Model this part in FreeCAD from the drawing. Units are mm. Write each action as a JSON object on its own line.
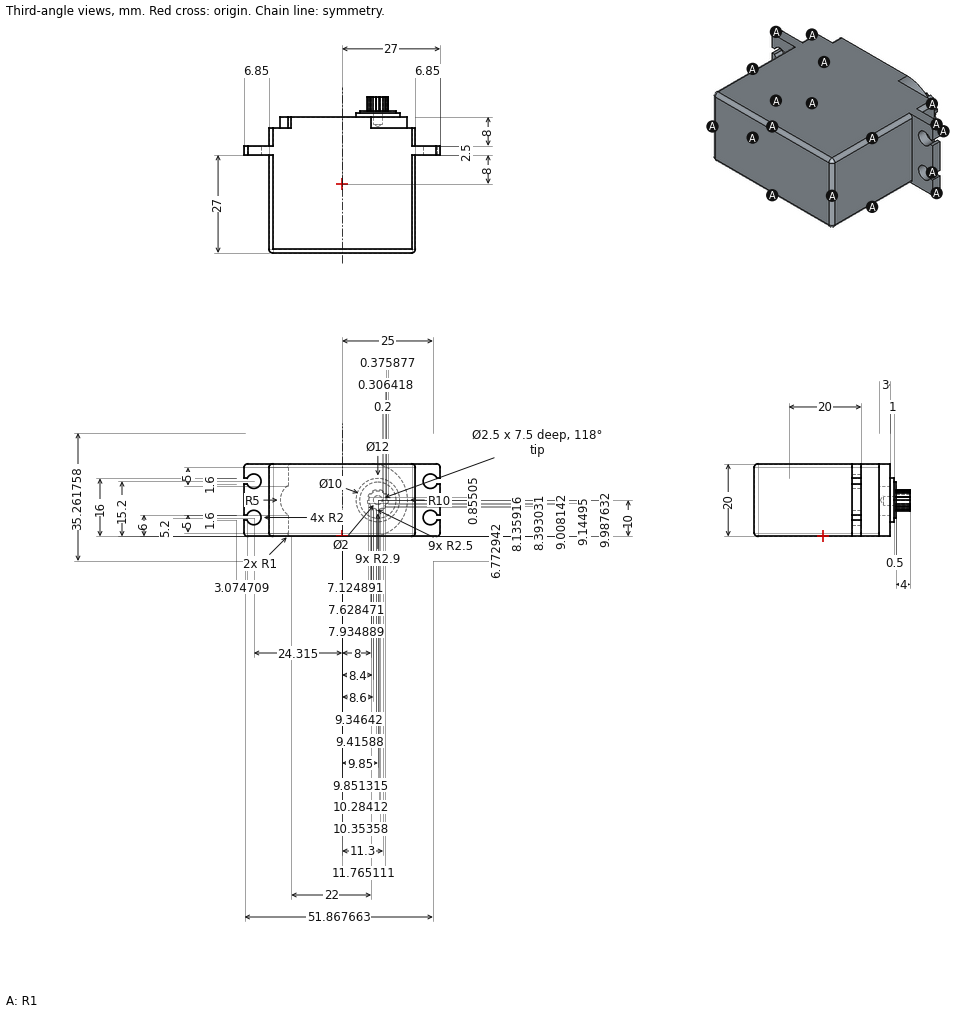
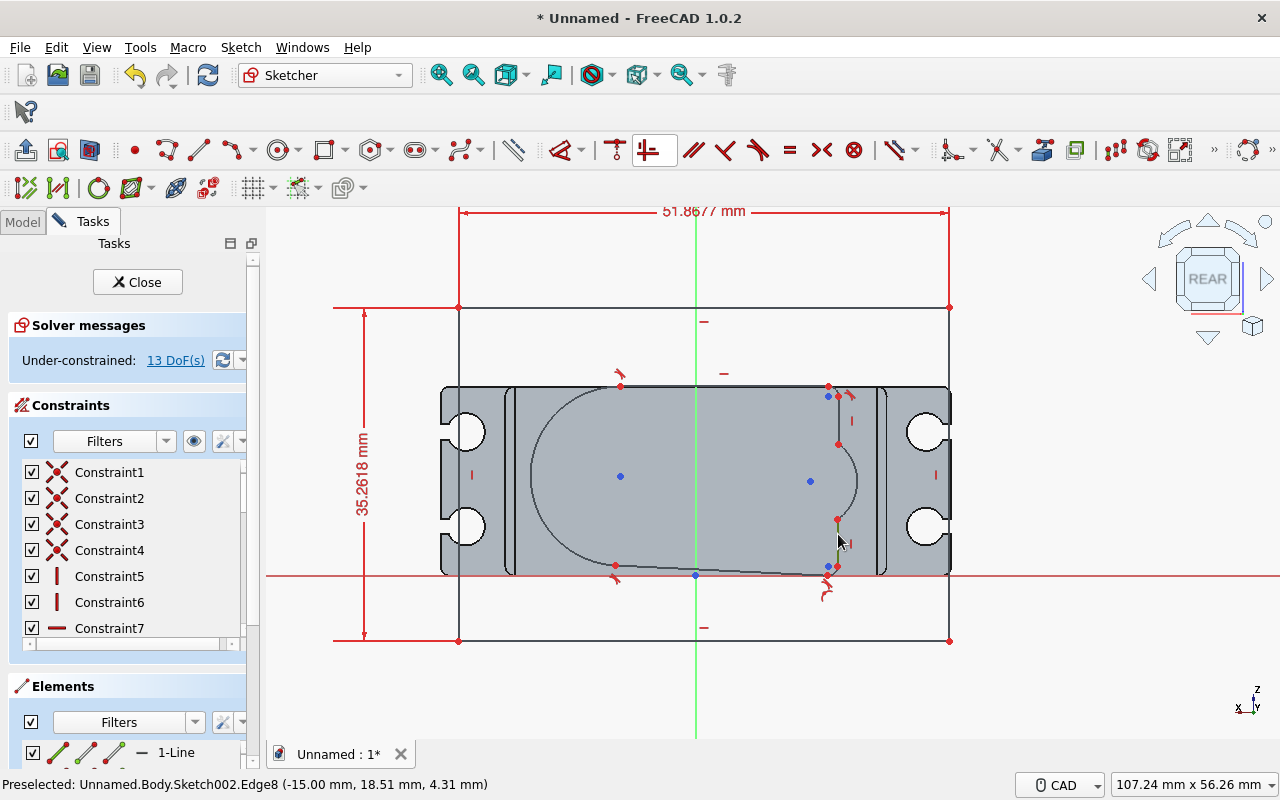
{"action": "scroll", "coordinate": [835, 573], "scroll_direction": "up", "scroll_amount": 4}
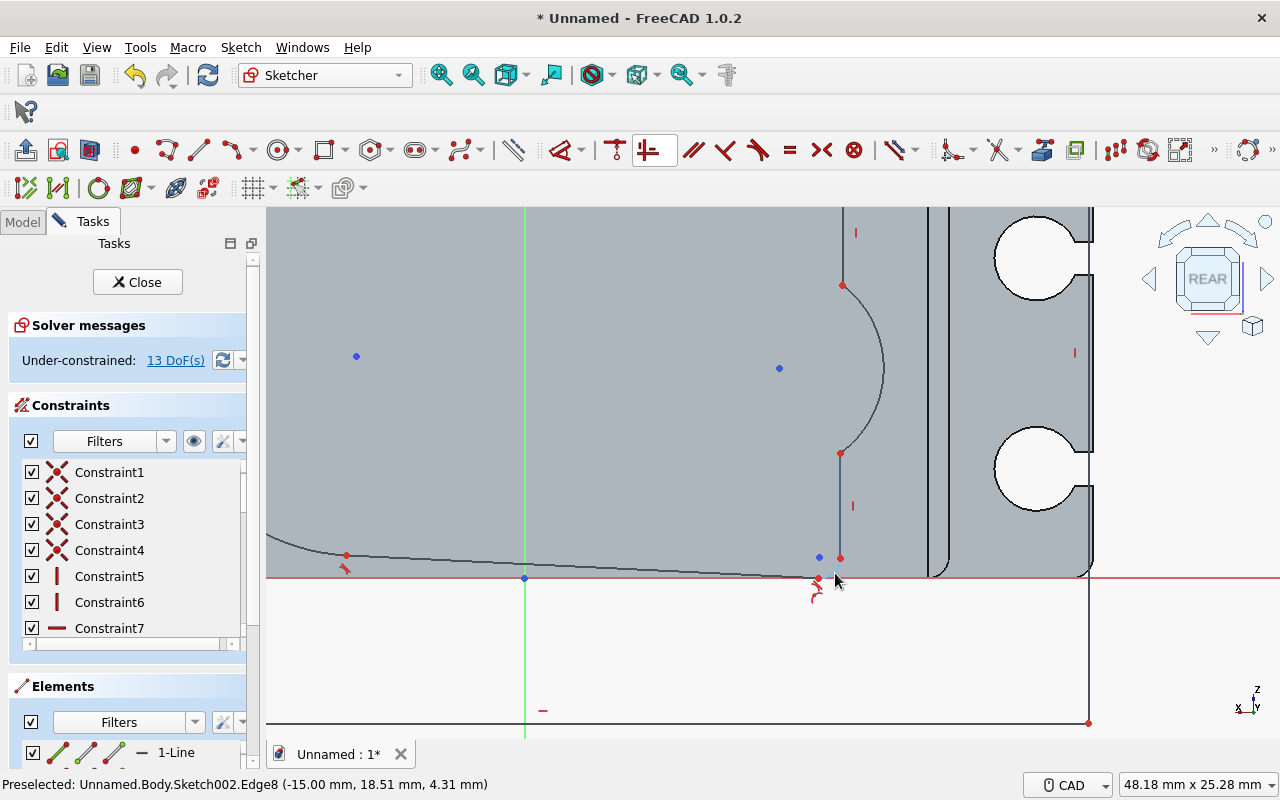
{"action": "left_click", "coordinate": [833, 573]}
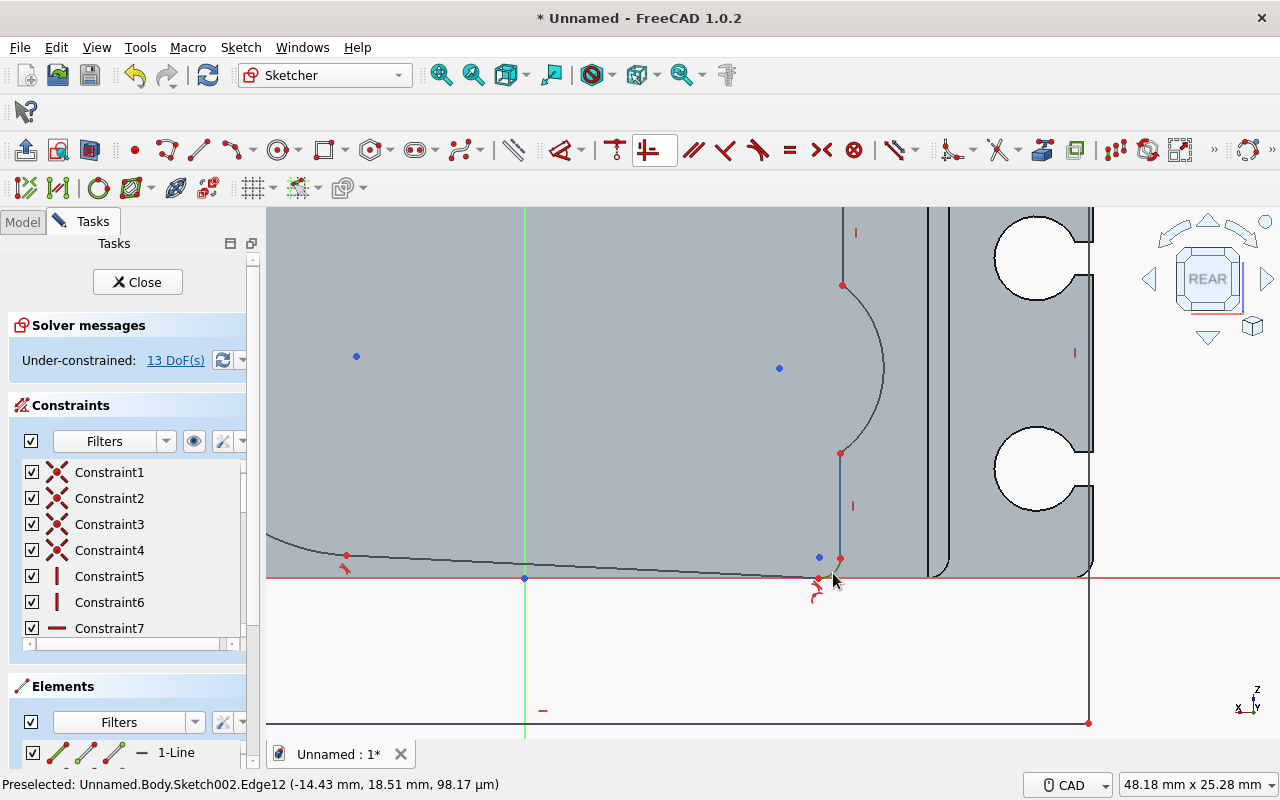
{"action": "left_click", "coordinate": [758, 150]}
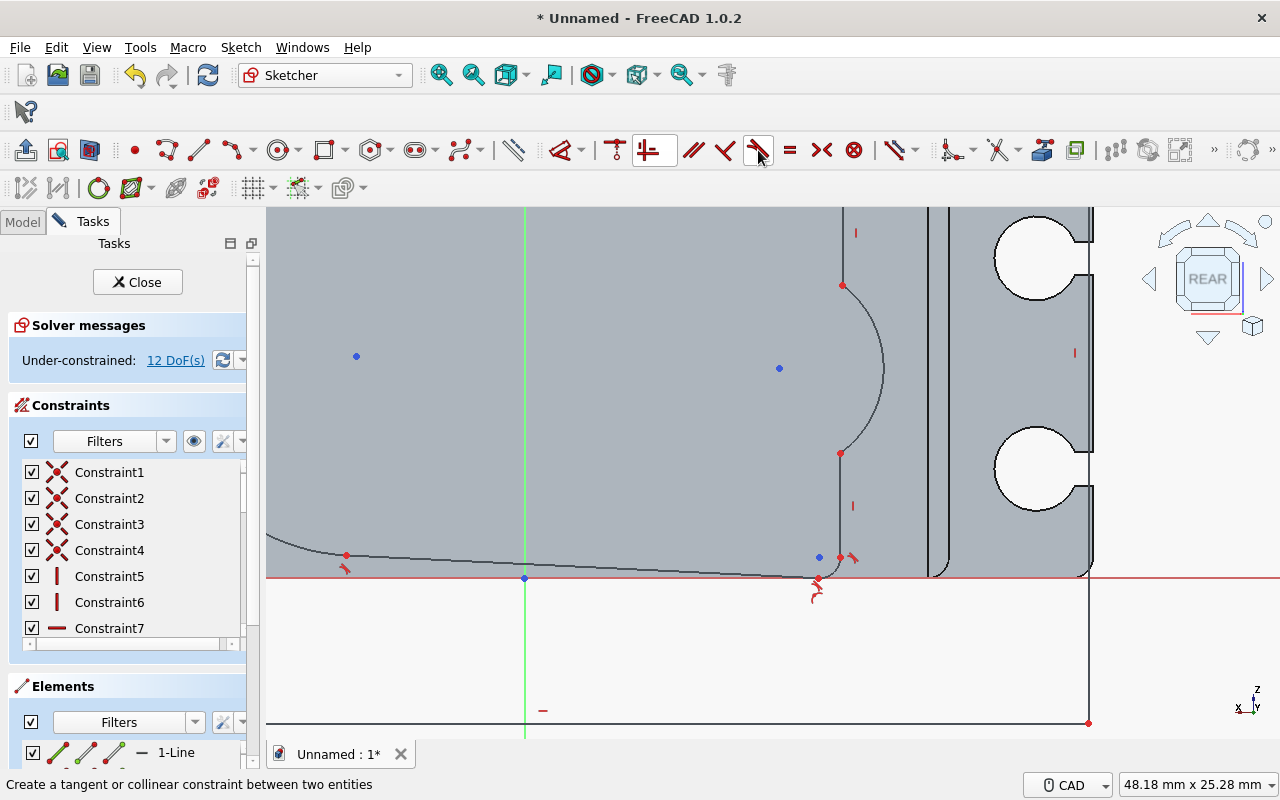
{"action": "left_click", "coordinate": [488, 562]}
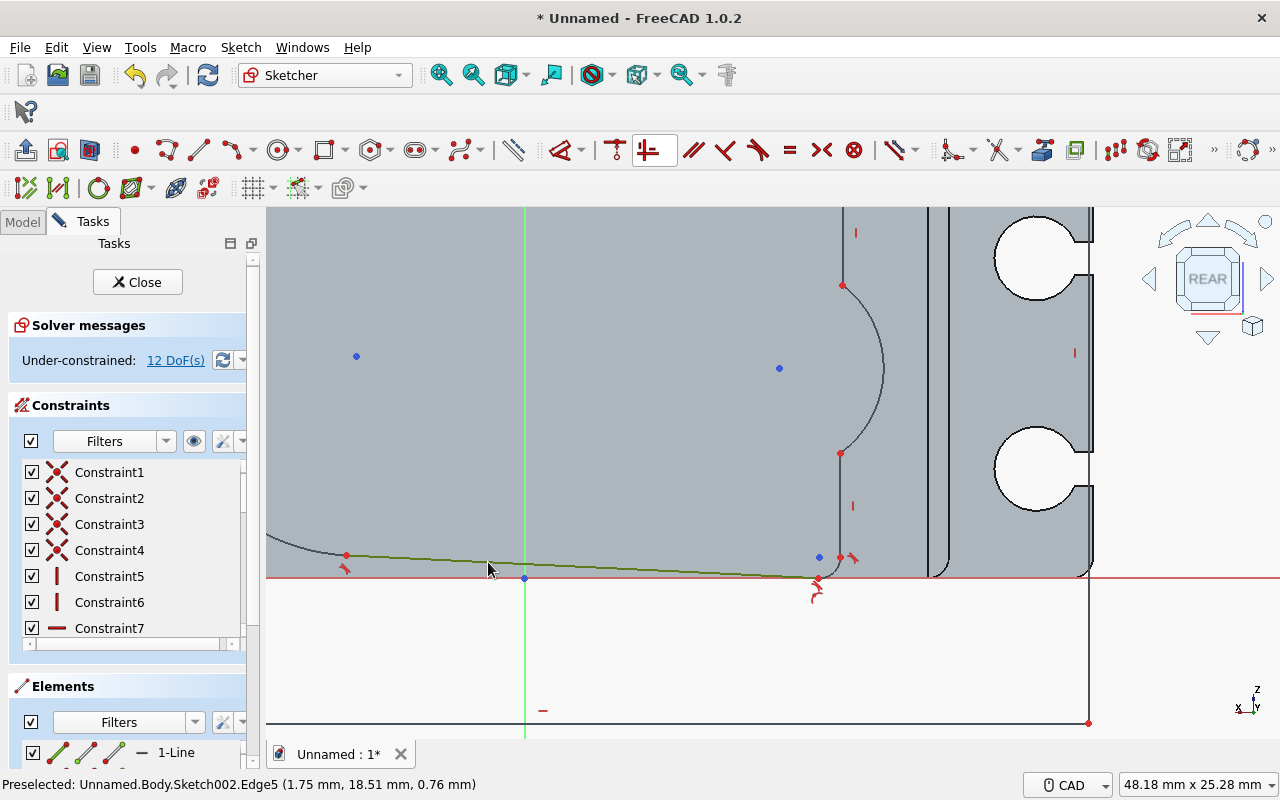
{"action": "key", "text": "h"}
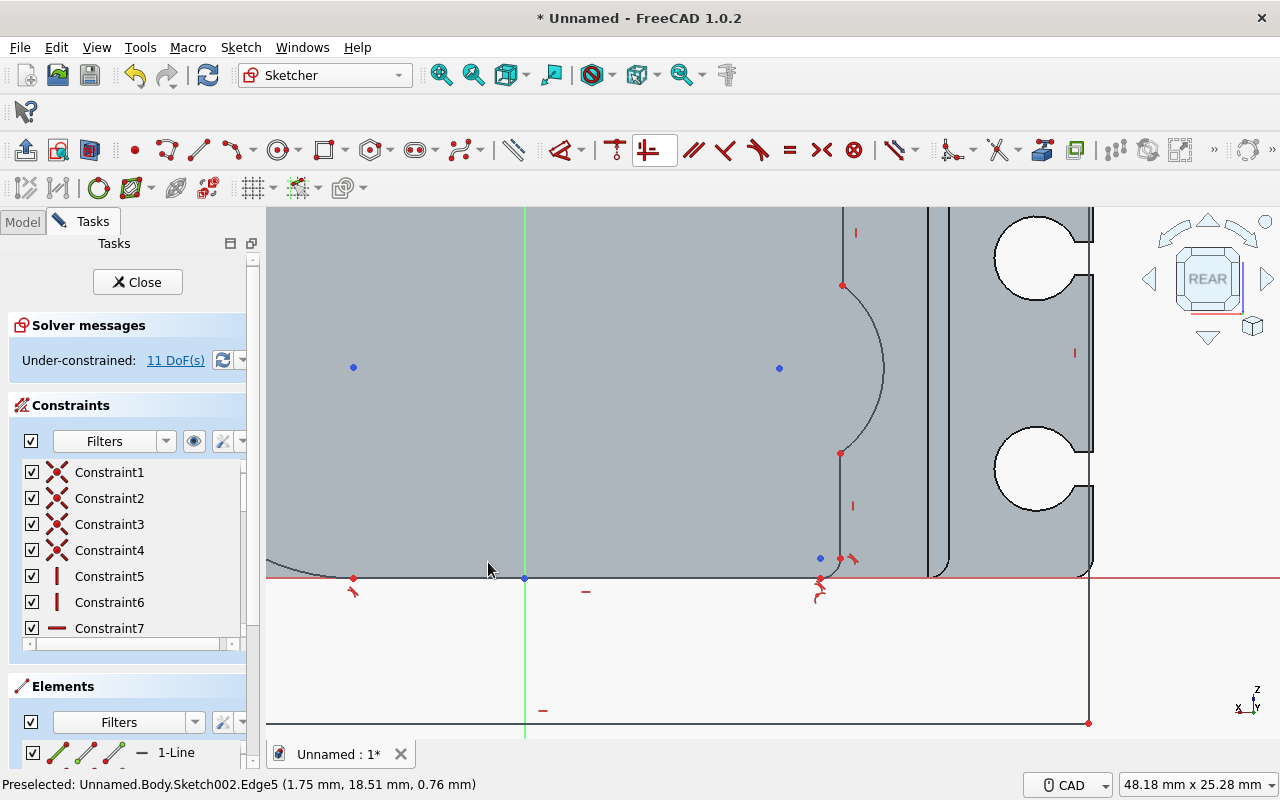
{"action": "scroll", "coordinate": [835, 574], "scroll_direction": "down", "scroll_amount": 4}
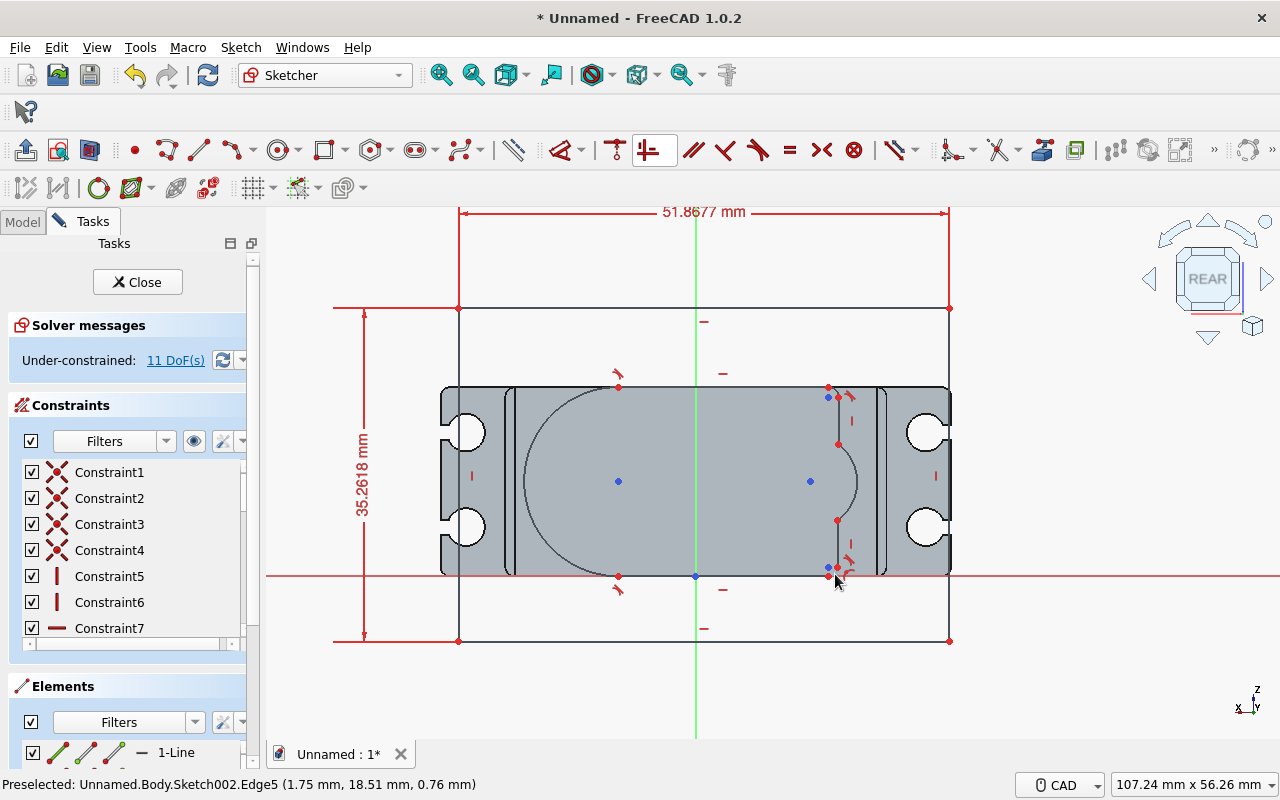
{"action": "scroll", "coordinate": [838, 393], "scroll_direction": "up", "scroll_amount": 6}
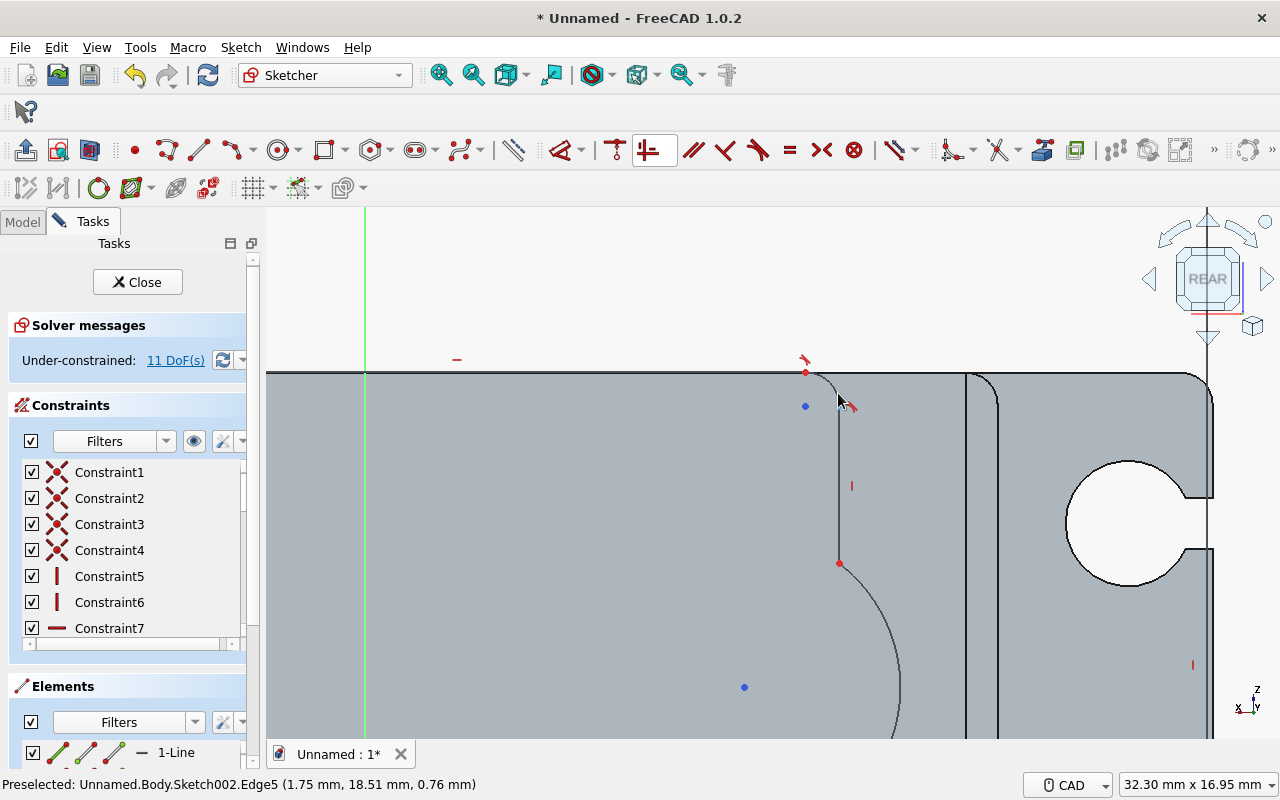
{"action": "left_click", "coordinate": [836, 391]}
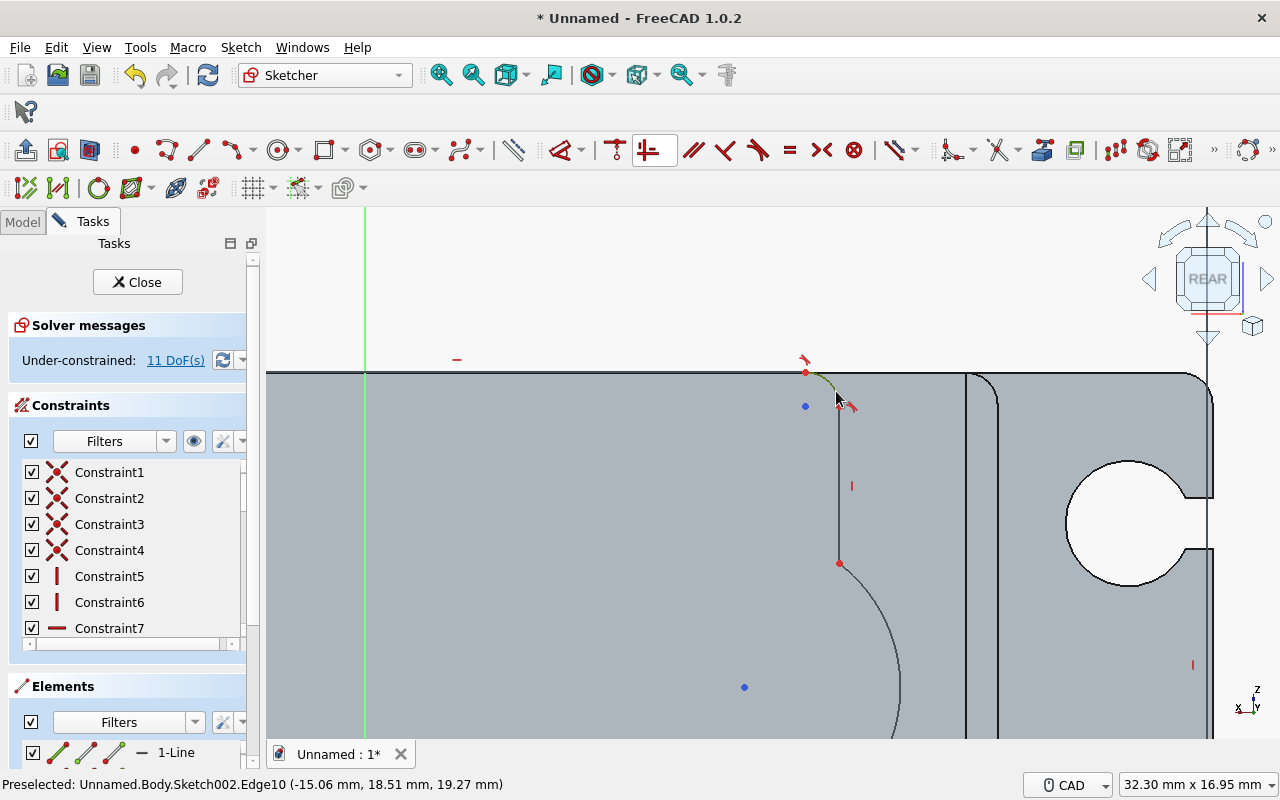
{"action": "scroll", "coordinate": [838, 392], "scroll_direction": "down", "scroll_amount": 6}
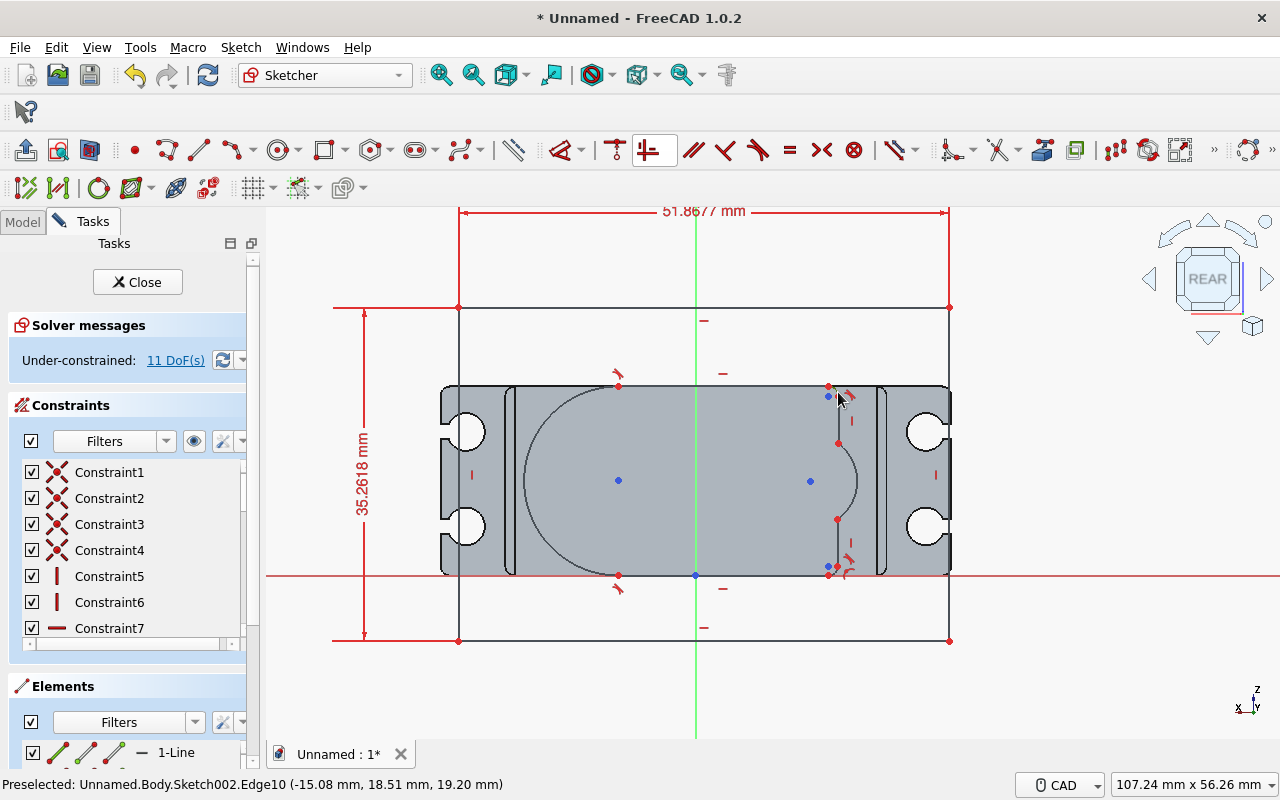
{"action": "scroll", "coordinate": [833, 575], "scroll_direction": "up", "scroll_amount": 6}